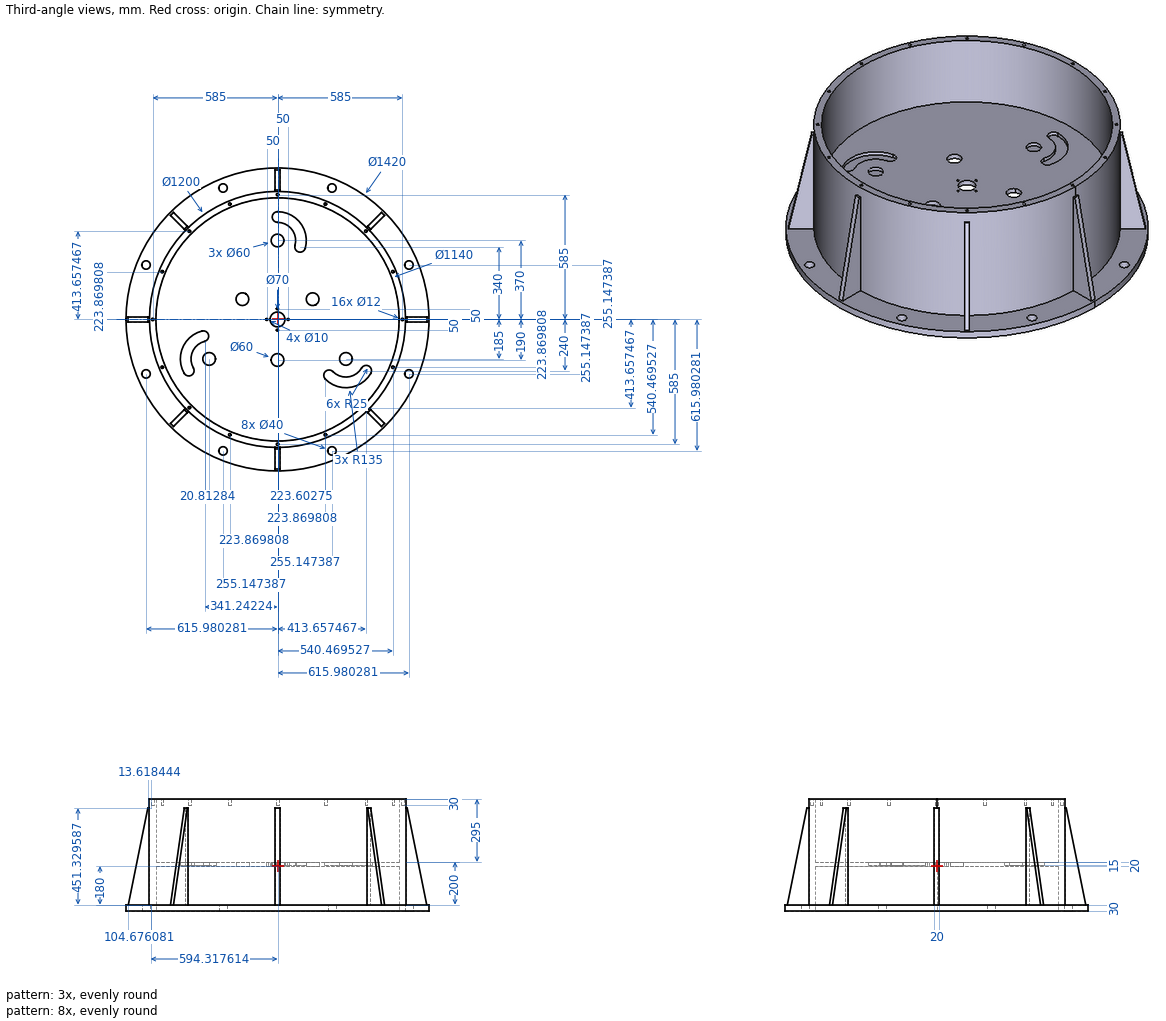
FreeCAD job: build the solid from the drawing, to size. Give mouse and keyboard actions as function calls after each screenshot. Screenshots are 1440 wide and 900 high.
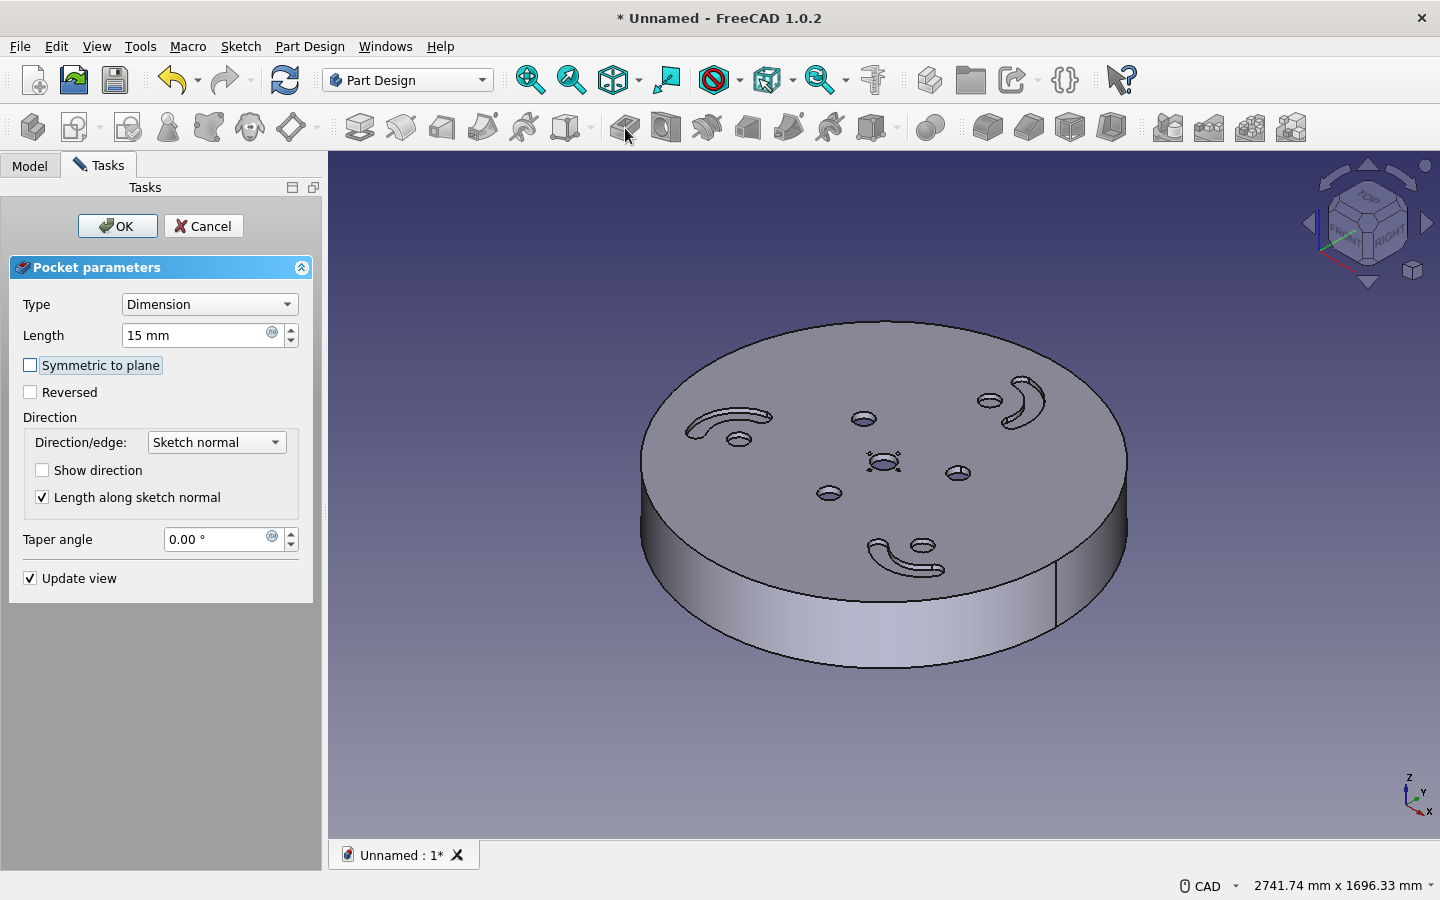
click(118, 226)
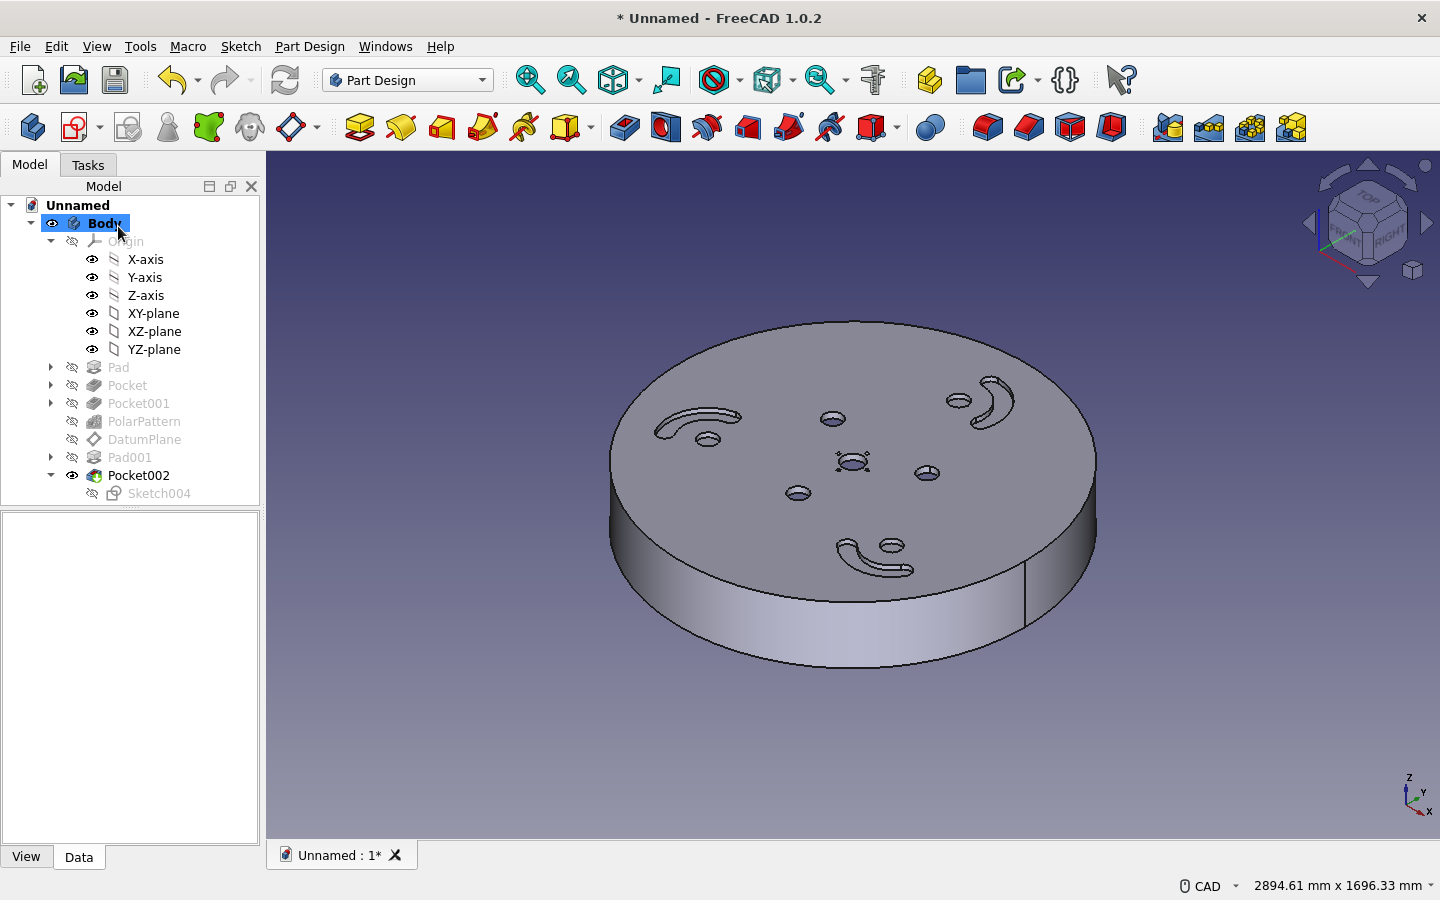
click(705, 489)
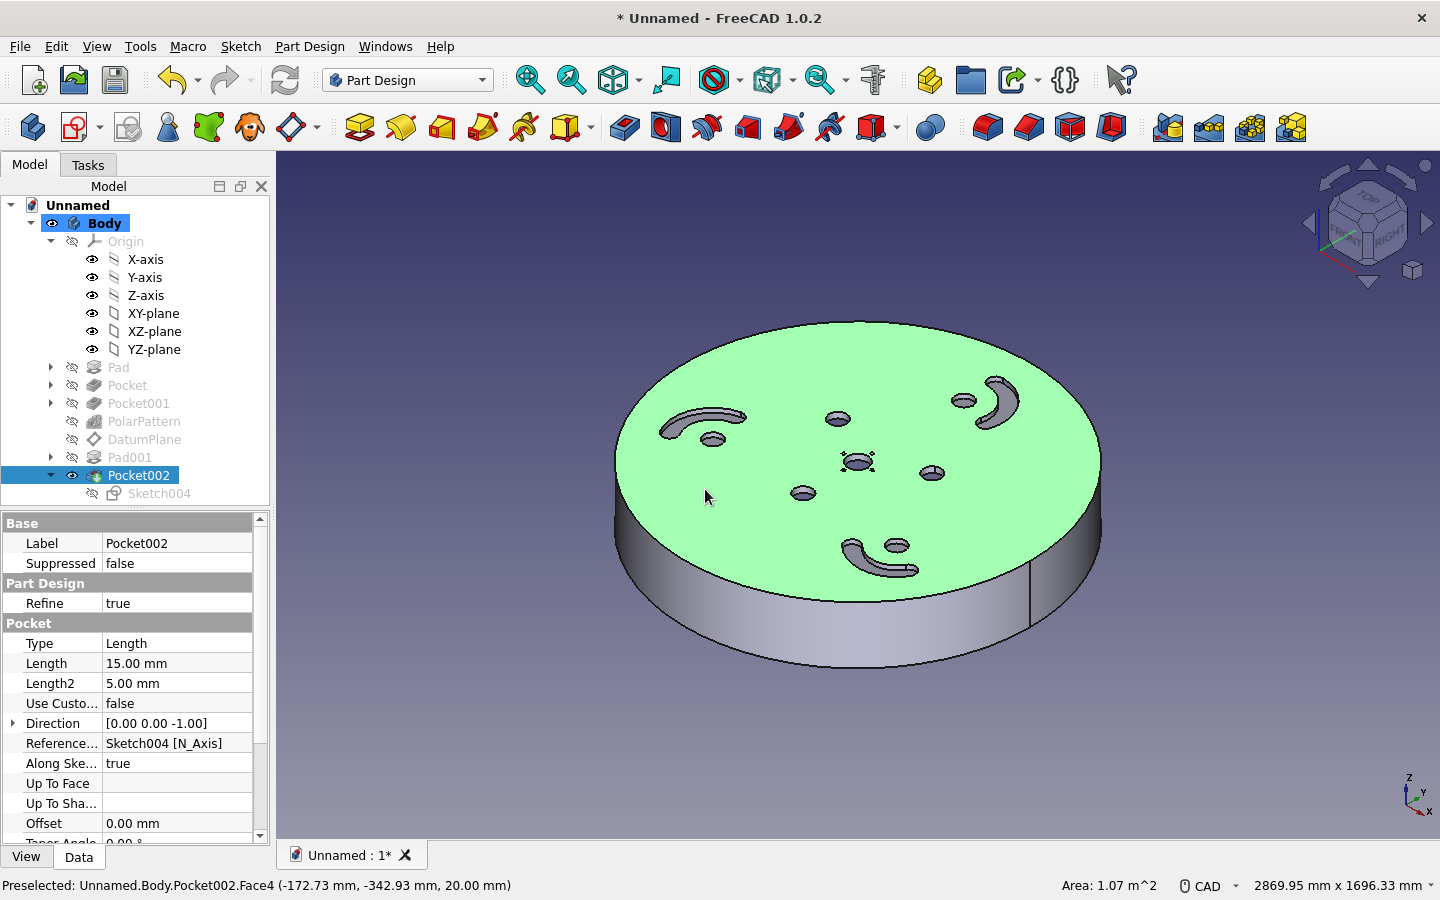
click(74, 128)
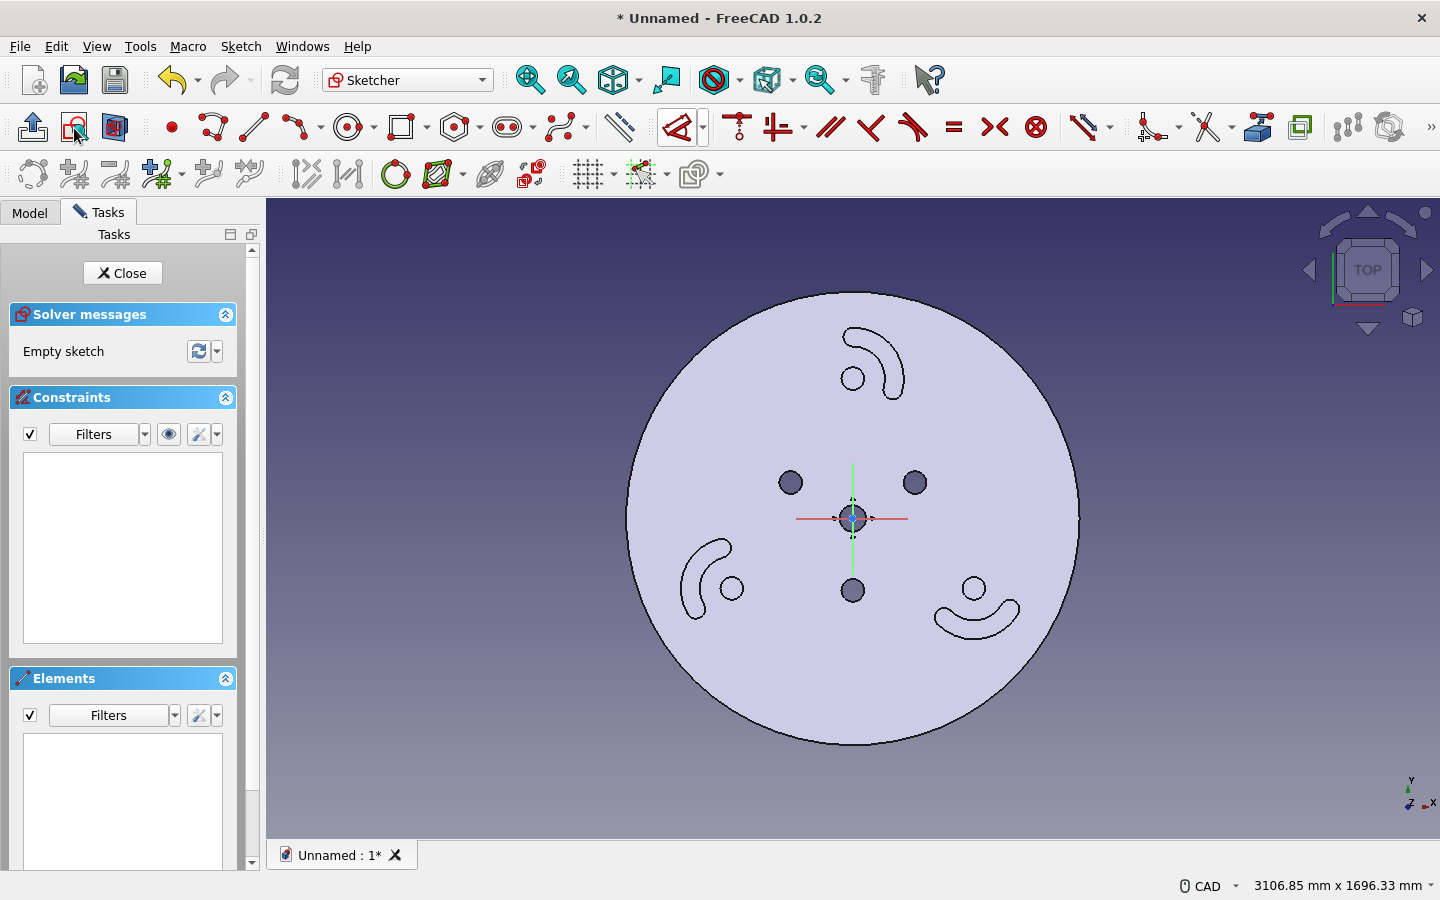
key(g)
key(c)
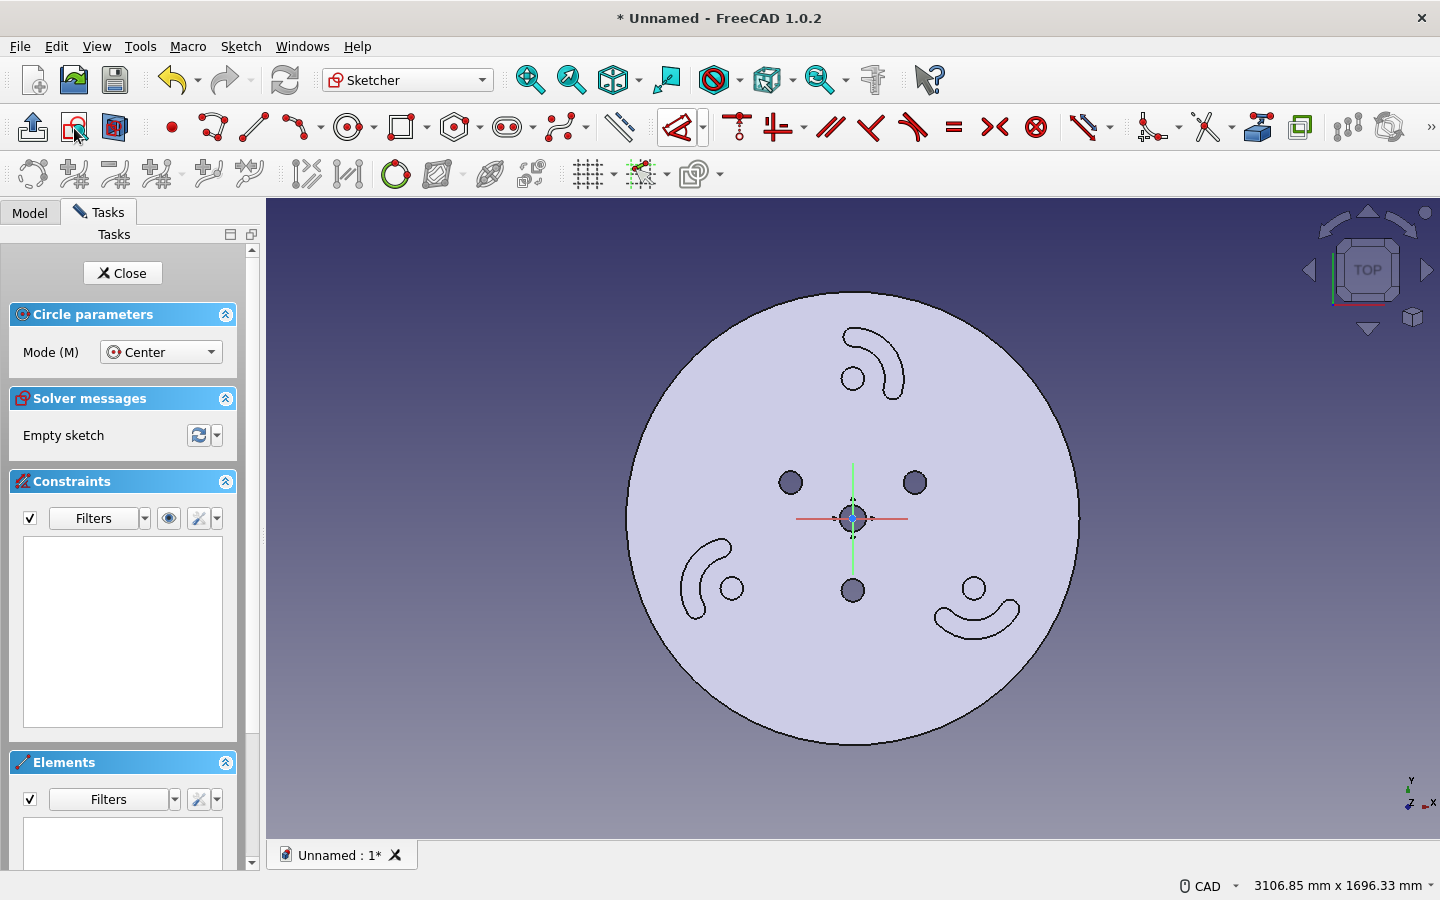
click(853, 518)
move(1013, 358)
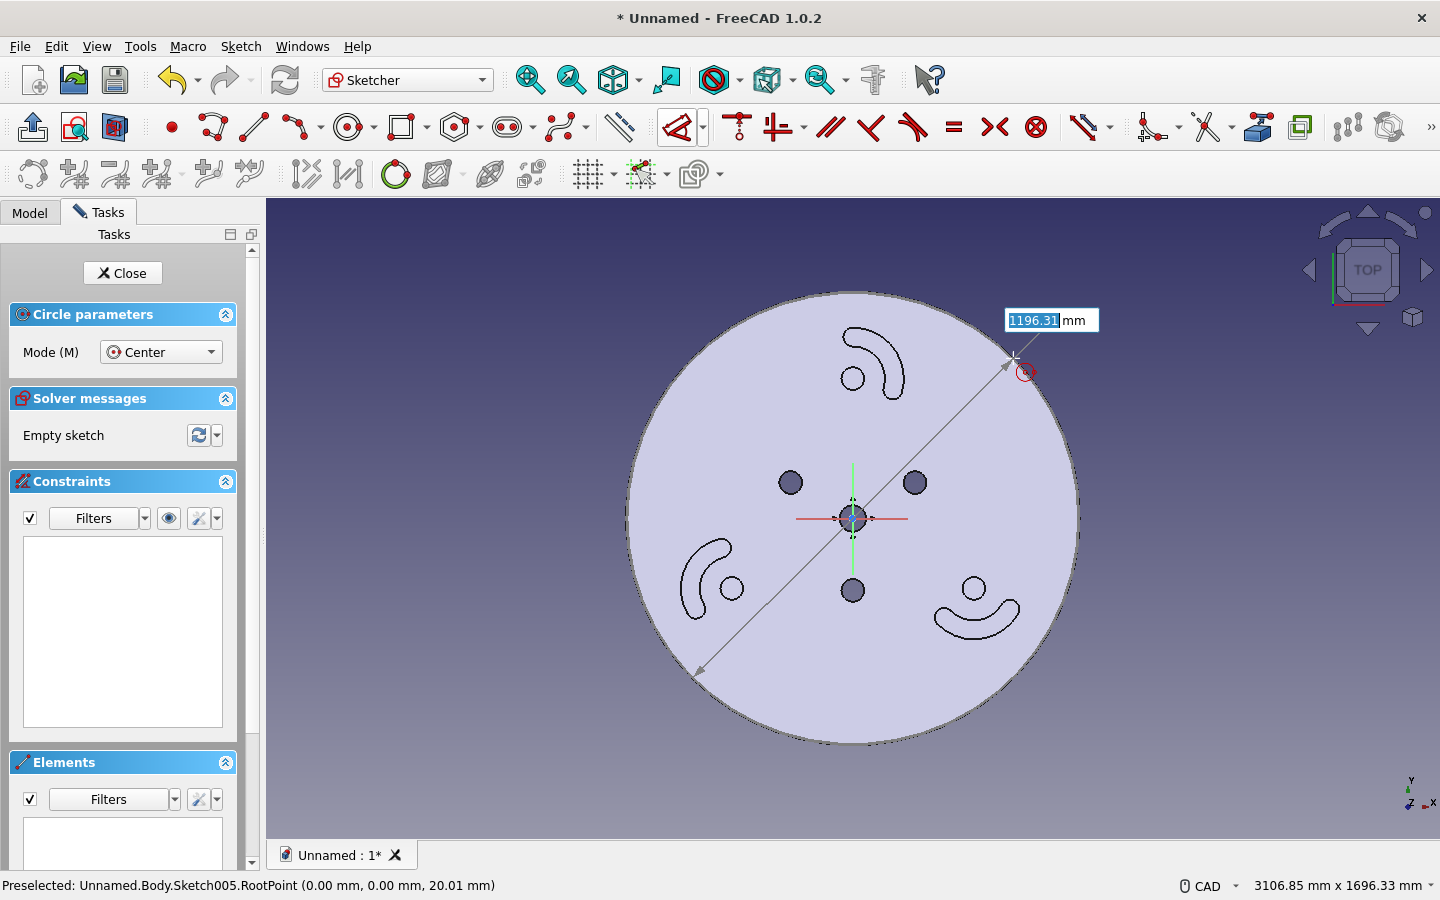
text(1200)
key(Return)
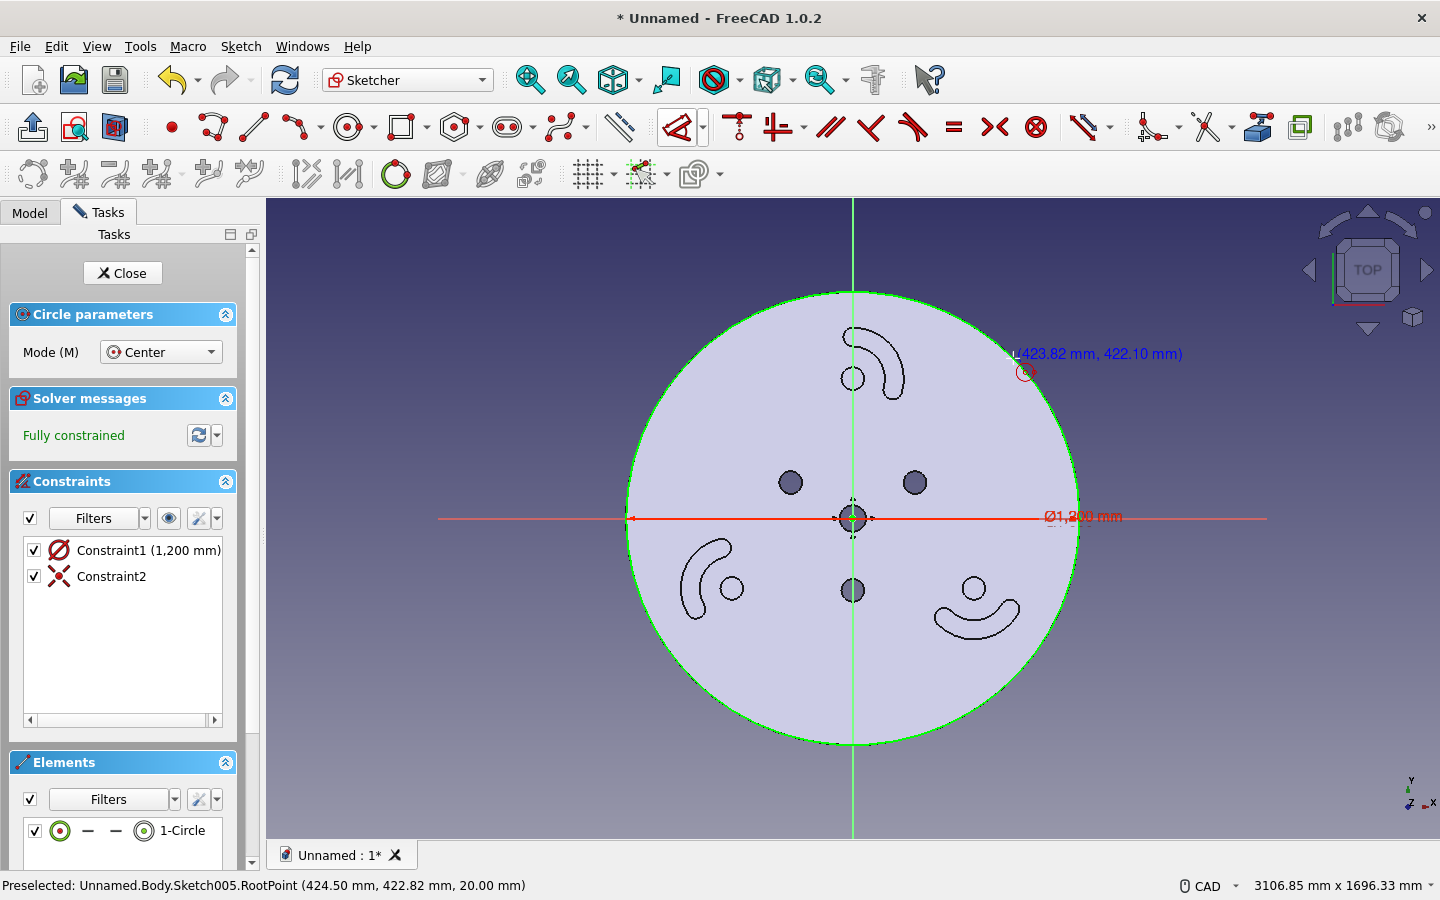
click(853, 518)